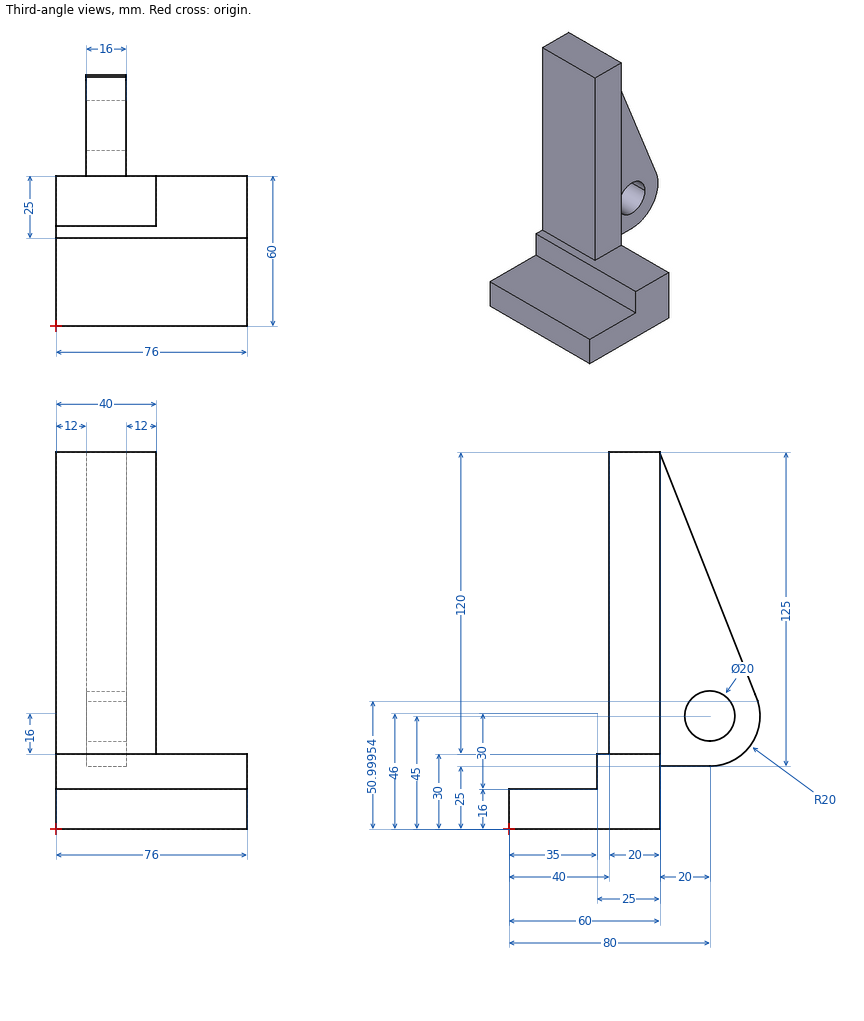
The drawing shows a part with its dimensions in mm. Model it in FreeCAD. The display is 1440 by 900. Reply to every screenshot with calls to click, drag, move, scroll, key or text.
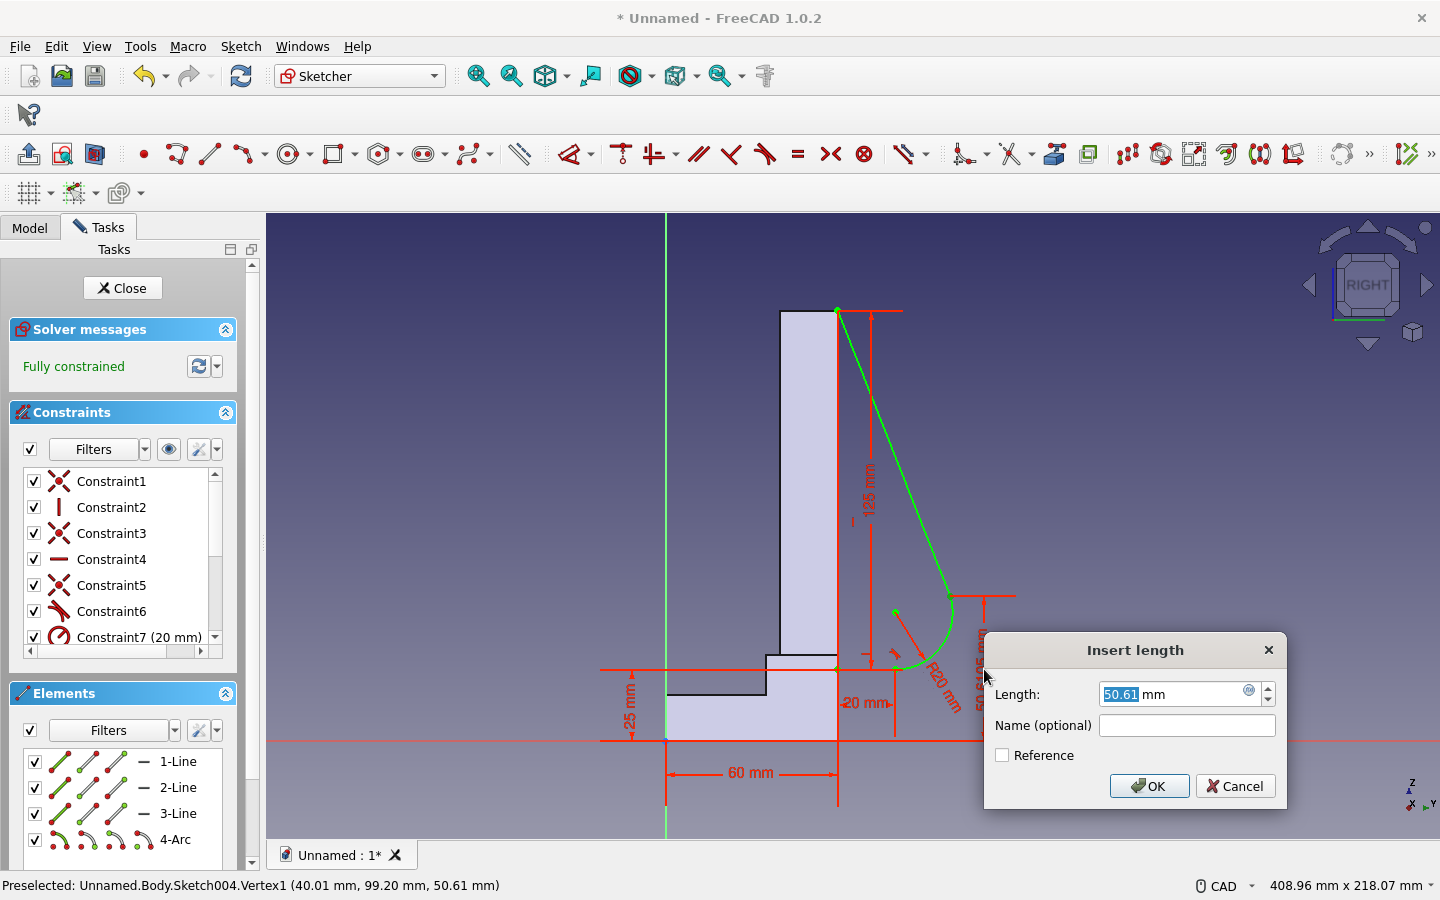
text(50.99954)
key(Return)
key(Escape)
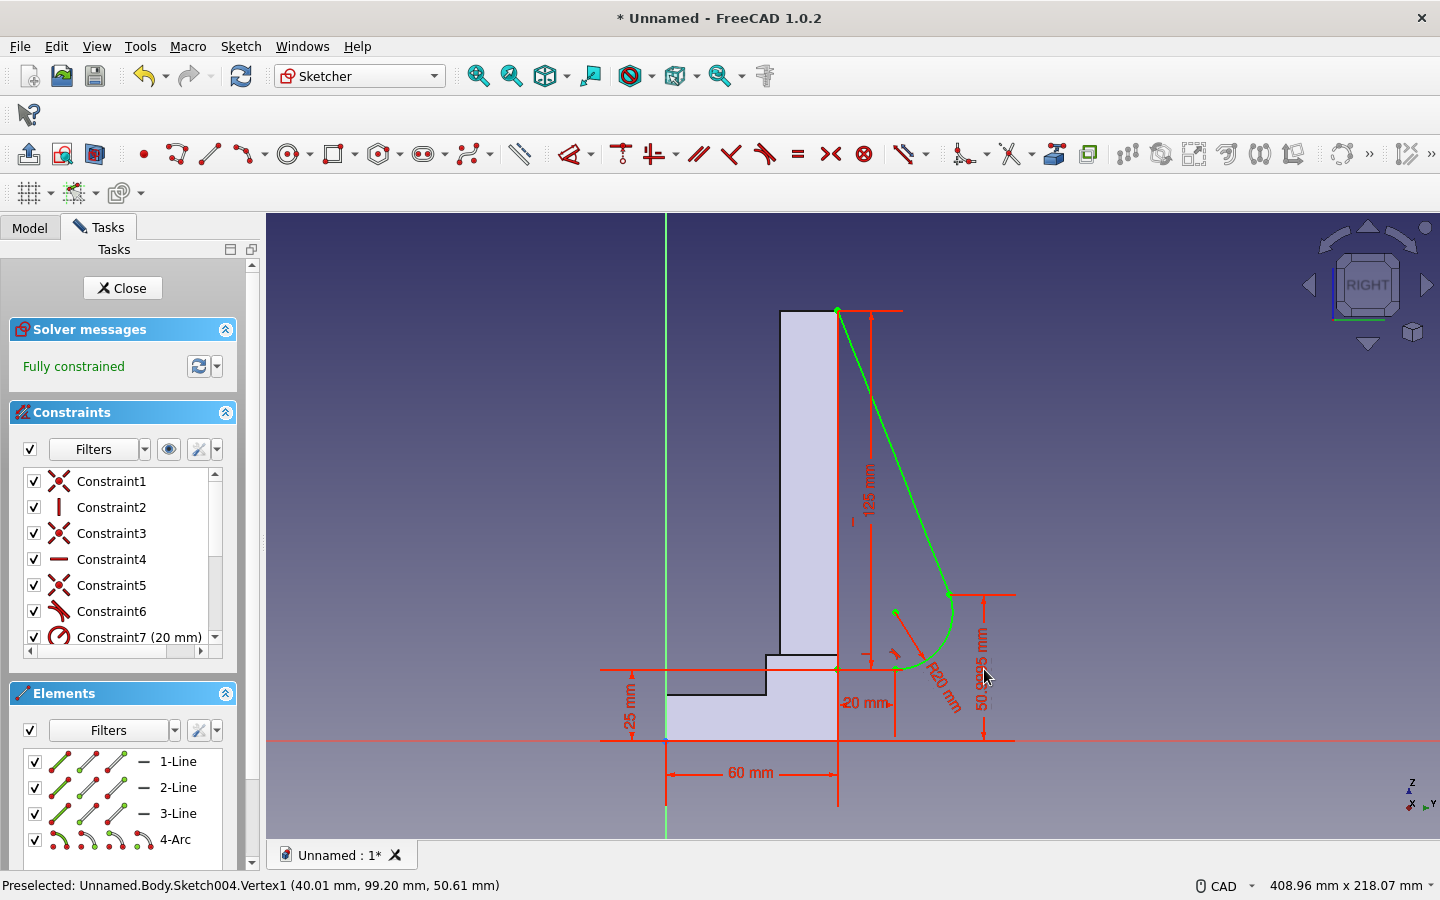
click(123, 288)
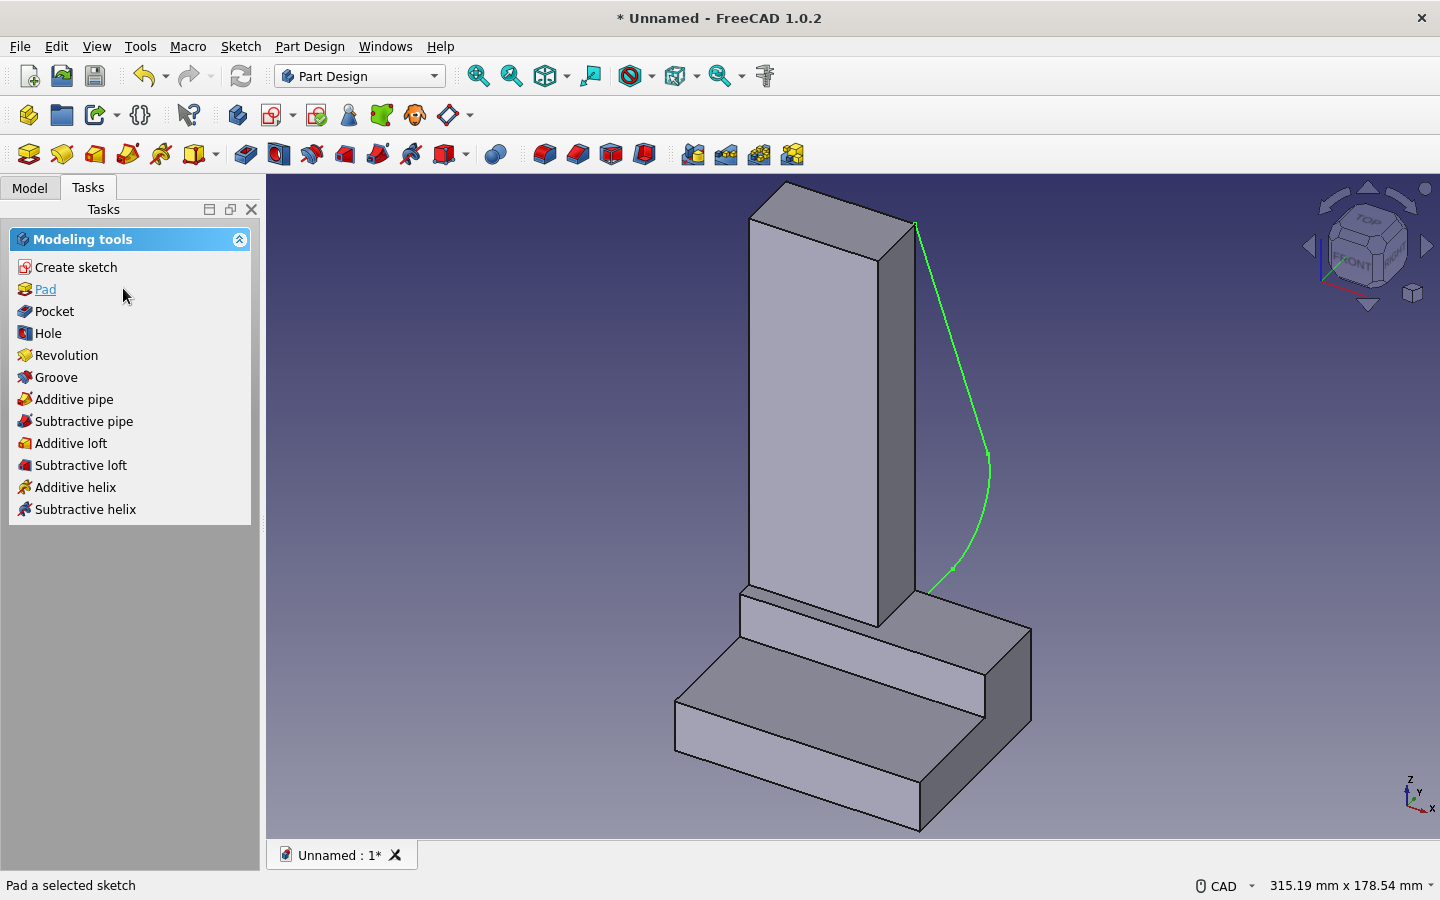
click(29, 154)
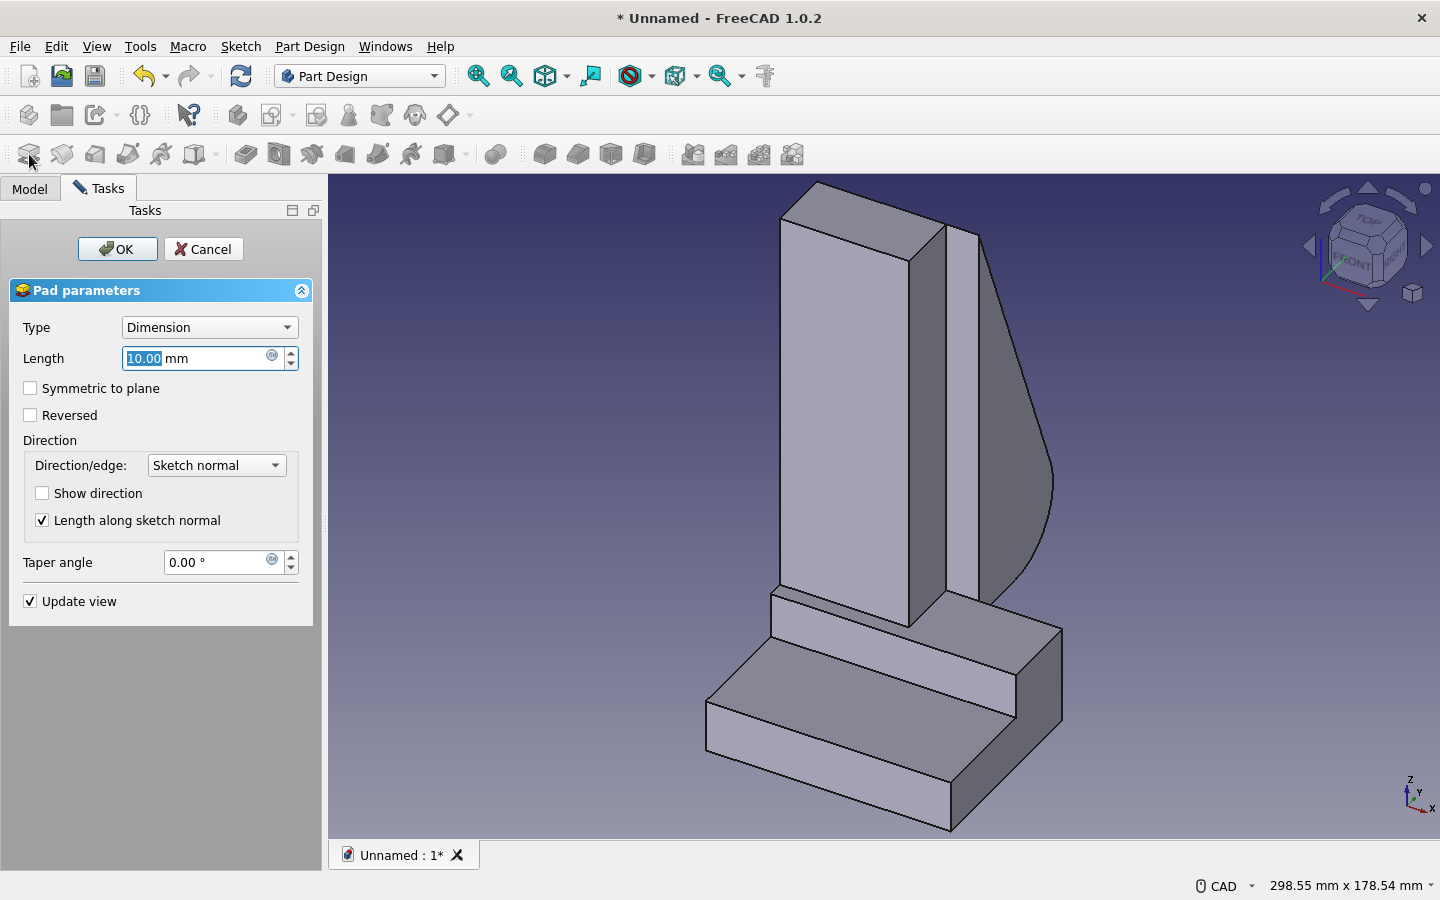
text(40)
key(Tab)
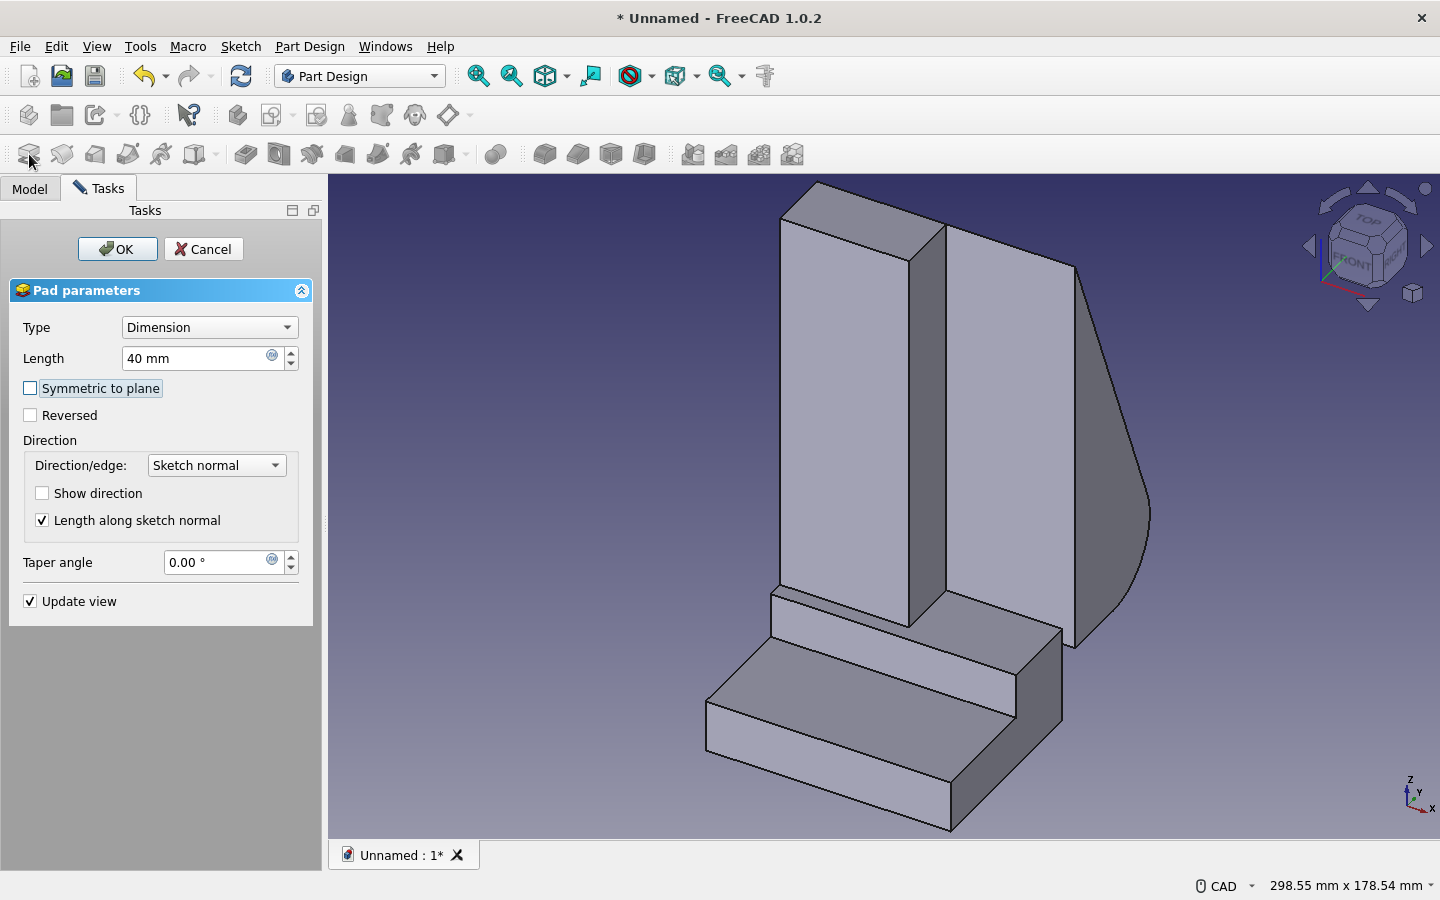
click(31, 415)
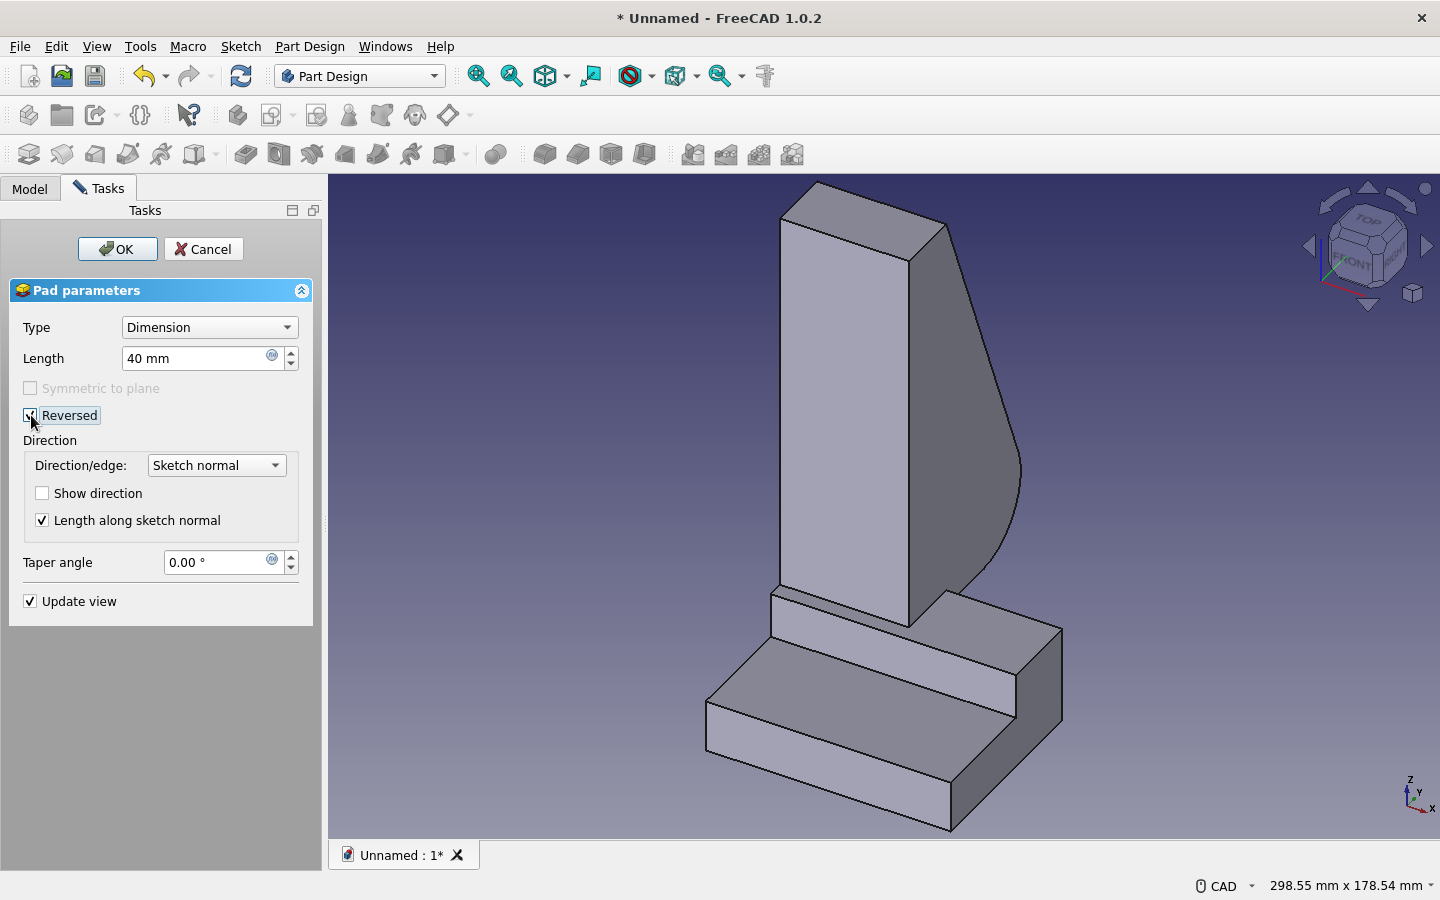
click(118, 249)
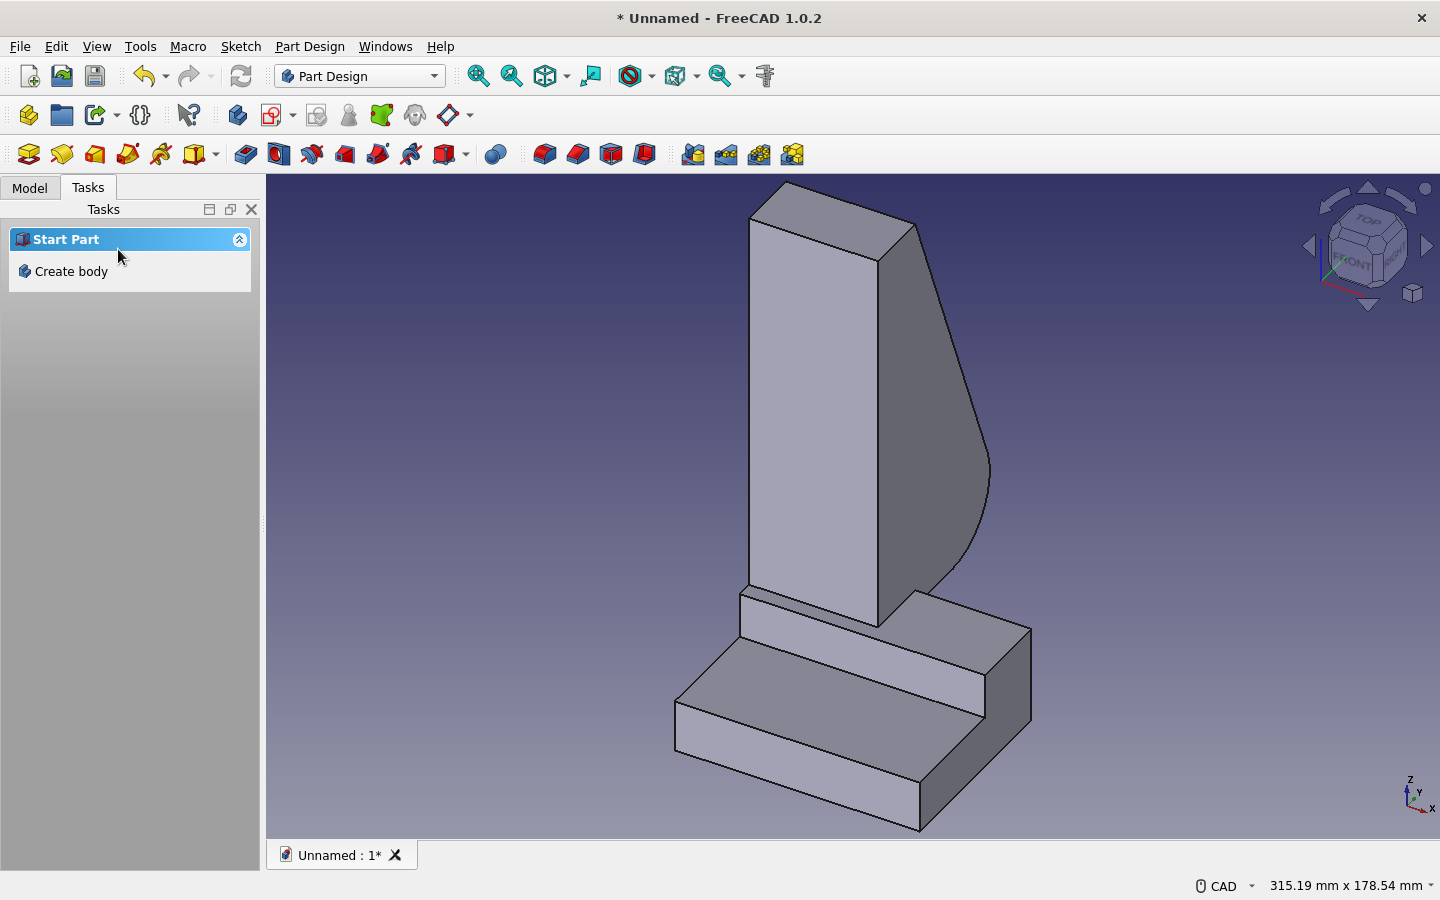
click(479, 76)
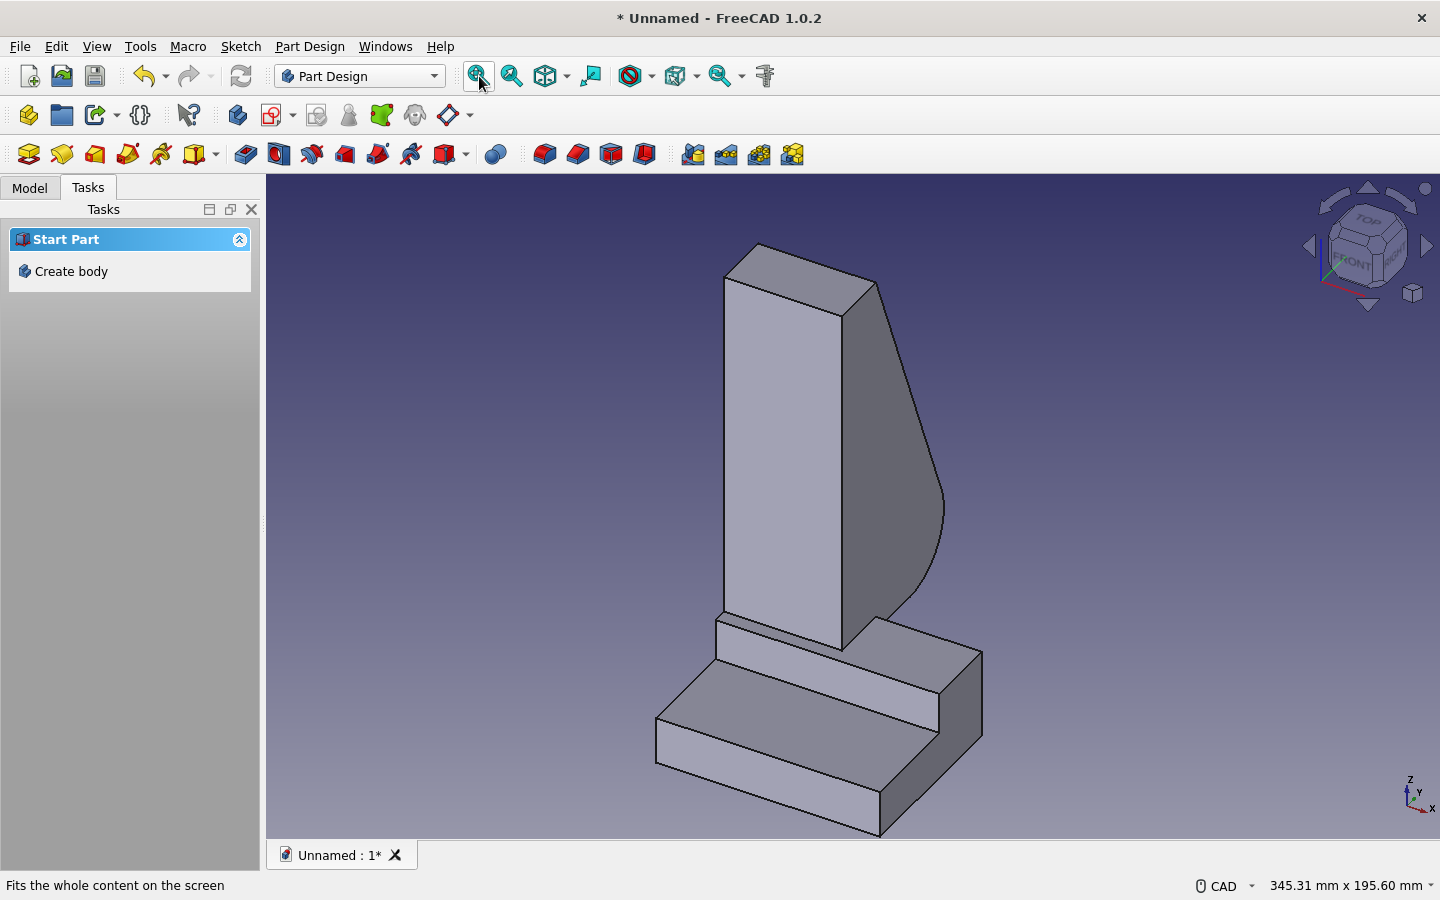
click(893, 538)